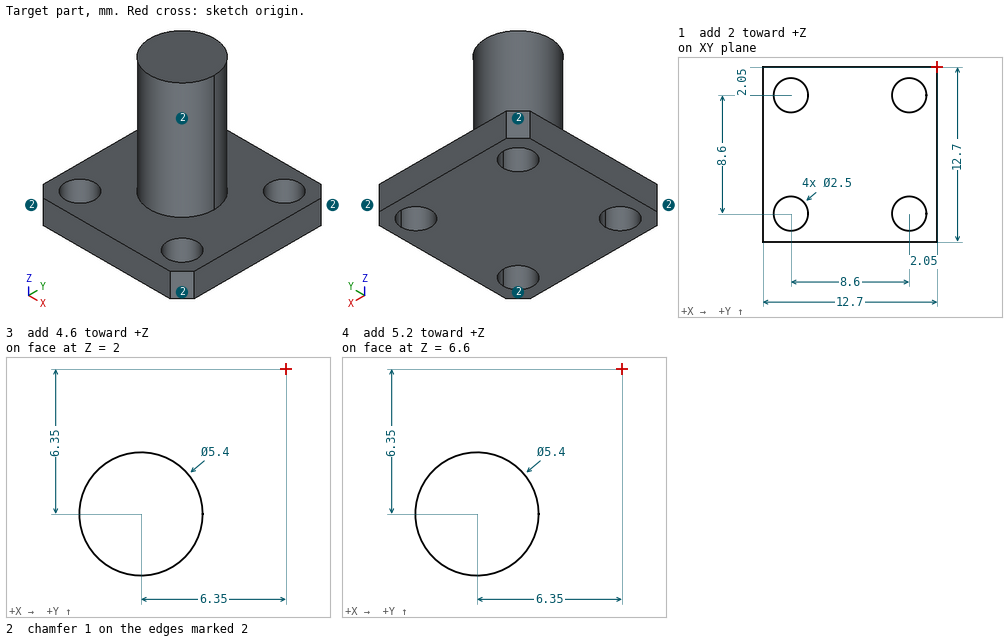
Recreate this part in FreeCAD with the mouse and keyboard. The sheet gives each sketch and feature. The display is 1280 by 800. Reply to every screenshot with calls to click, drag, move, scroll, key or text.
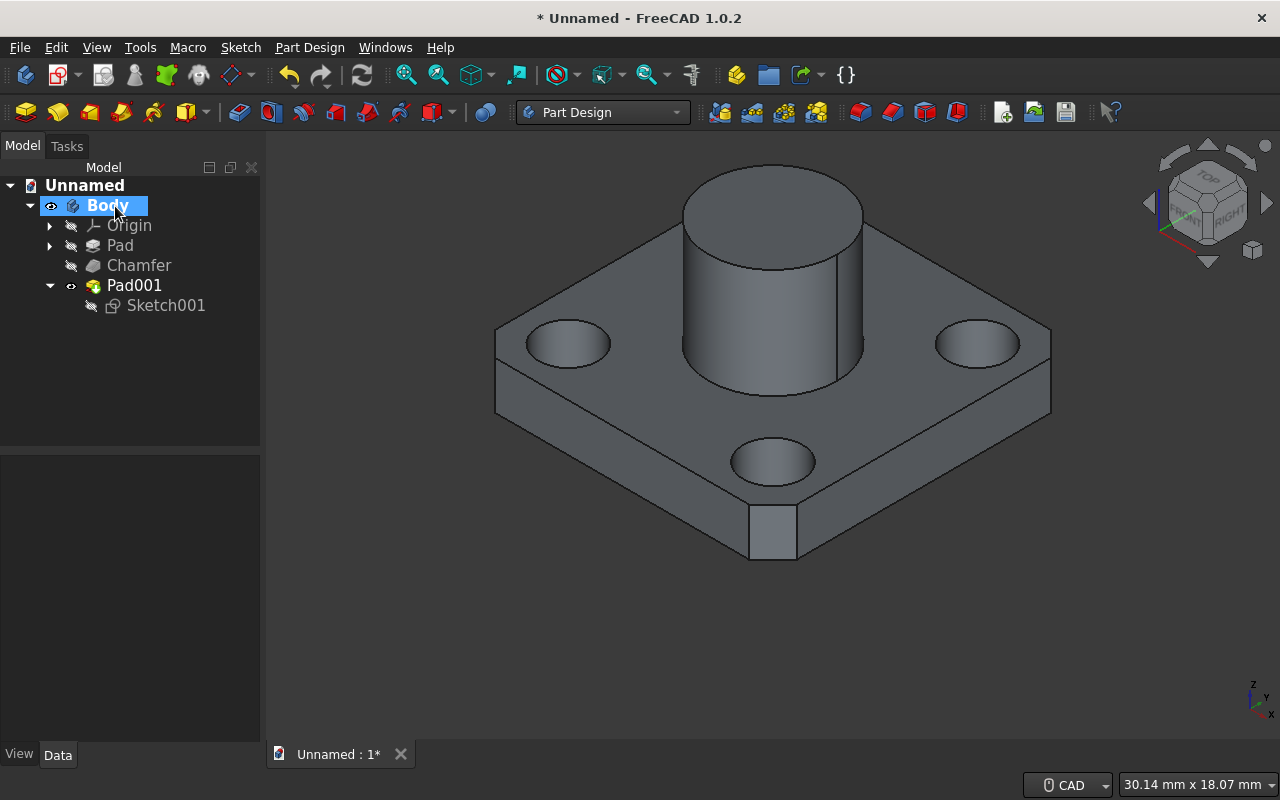
key(v)
key(f)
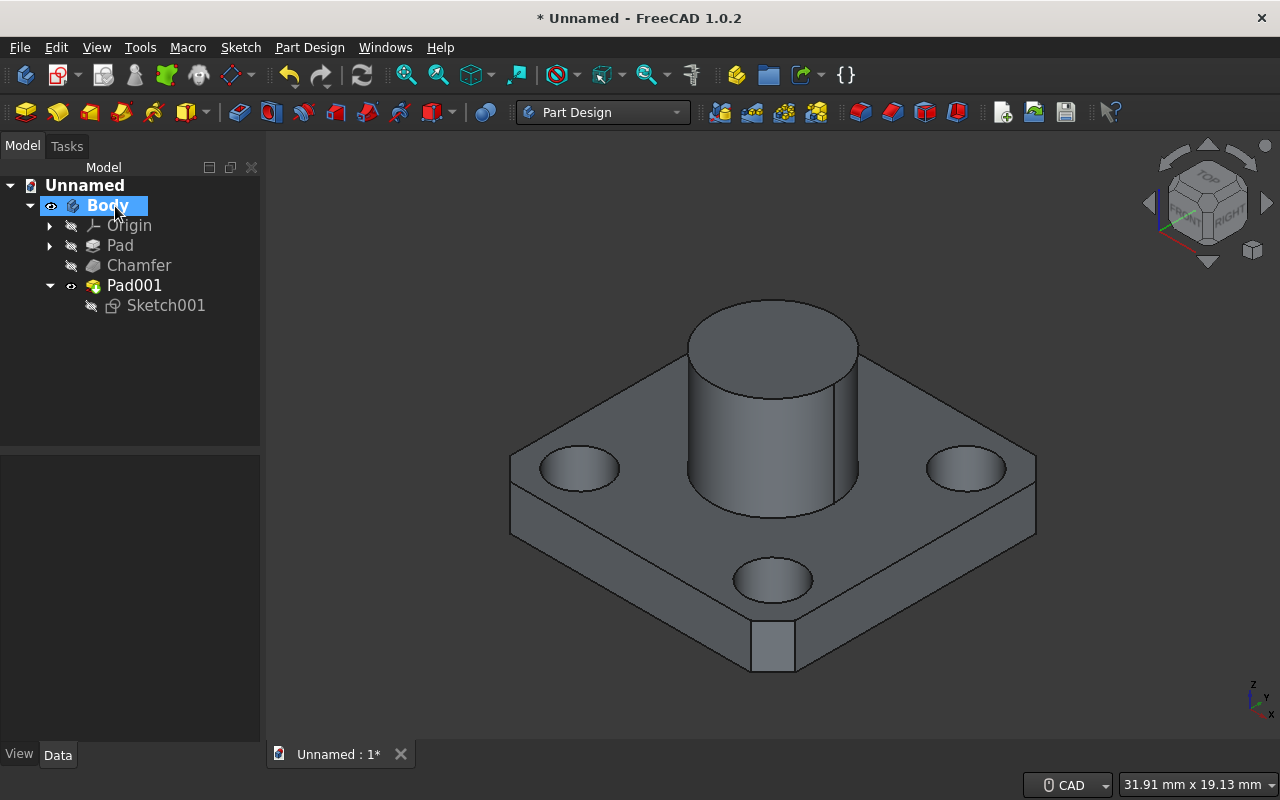
click(773, 348)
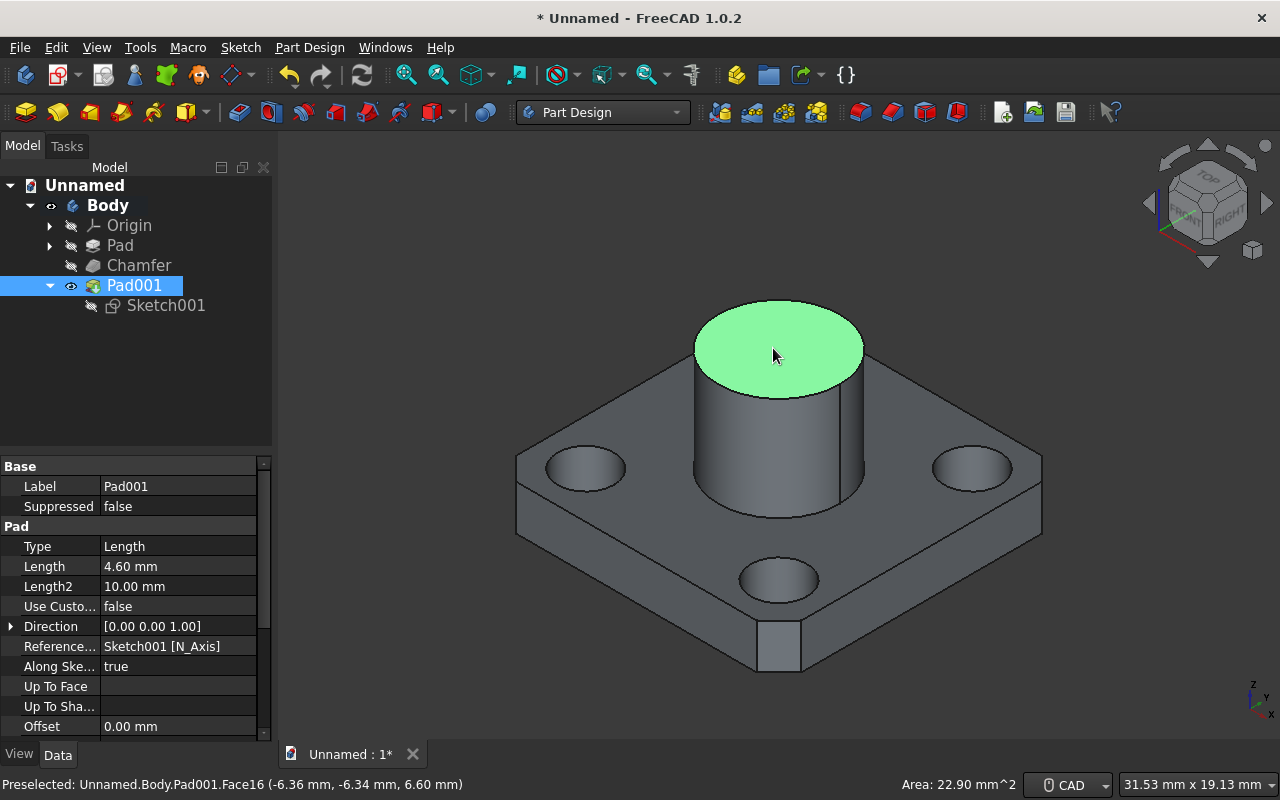
click(58, 76)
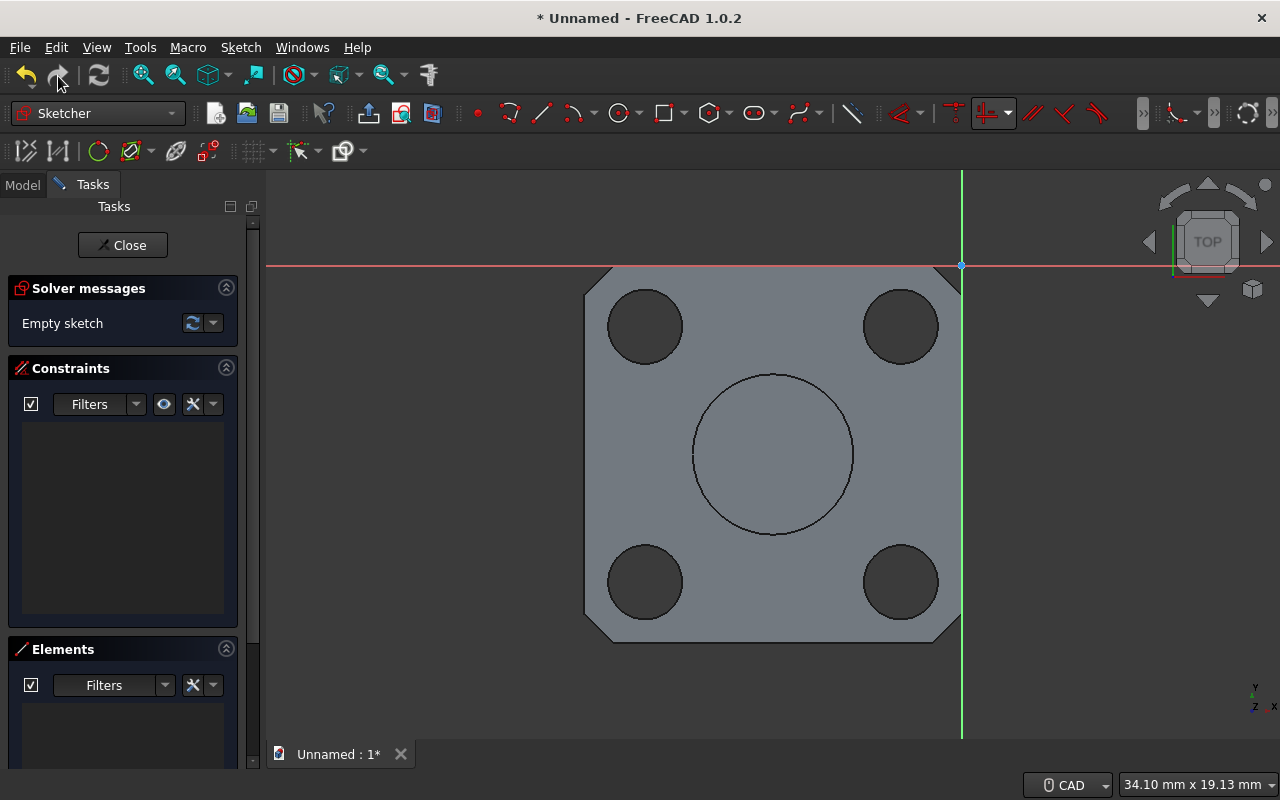
key(g)
key(c)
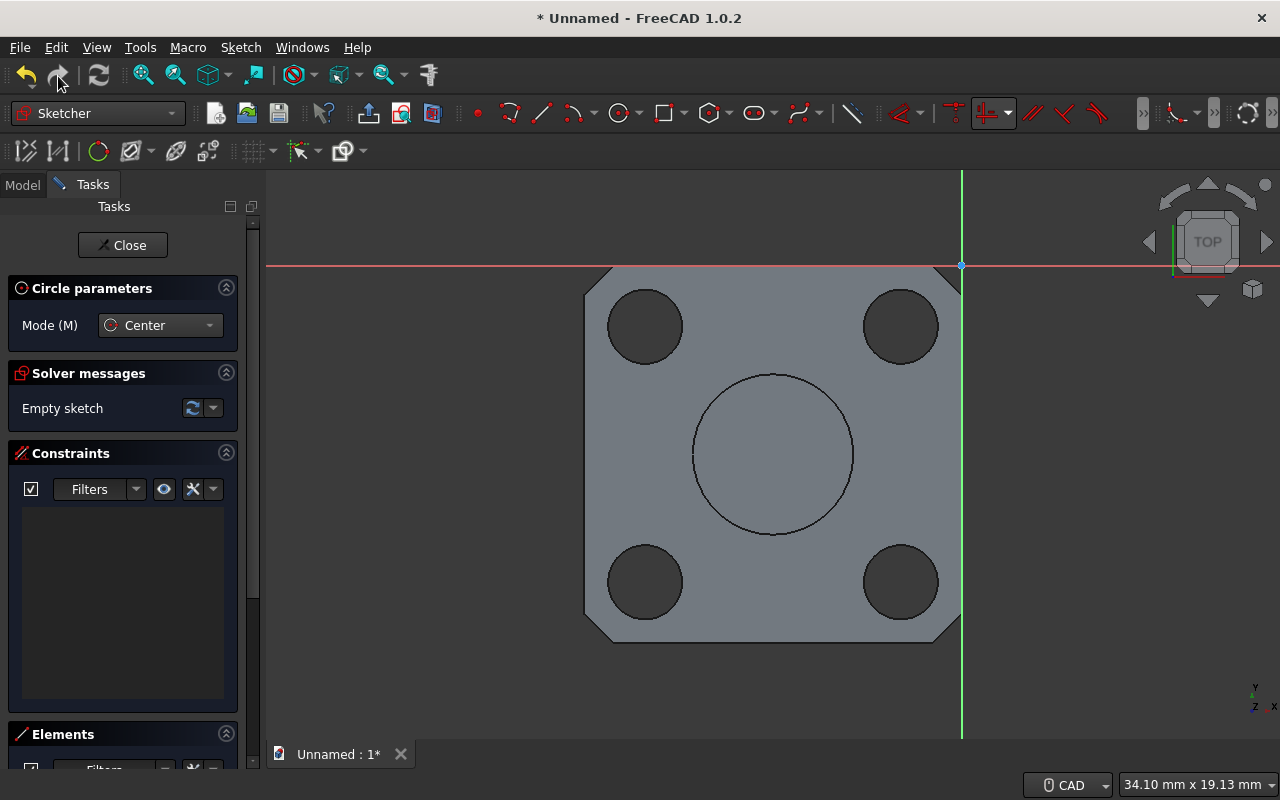
click(773, 455)
move(830, 398)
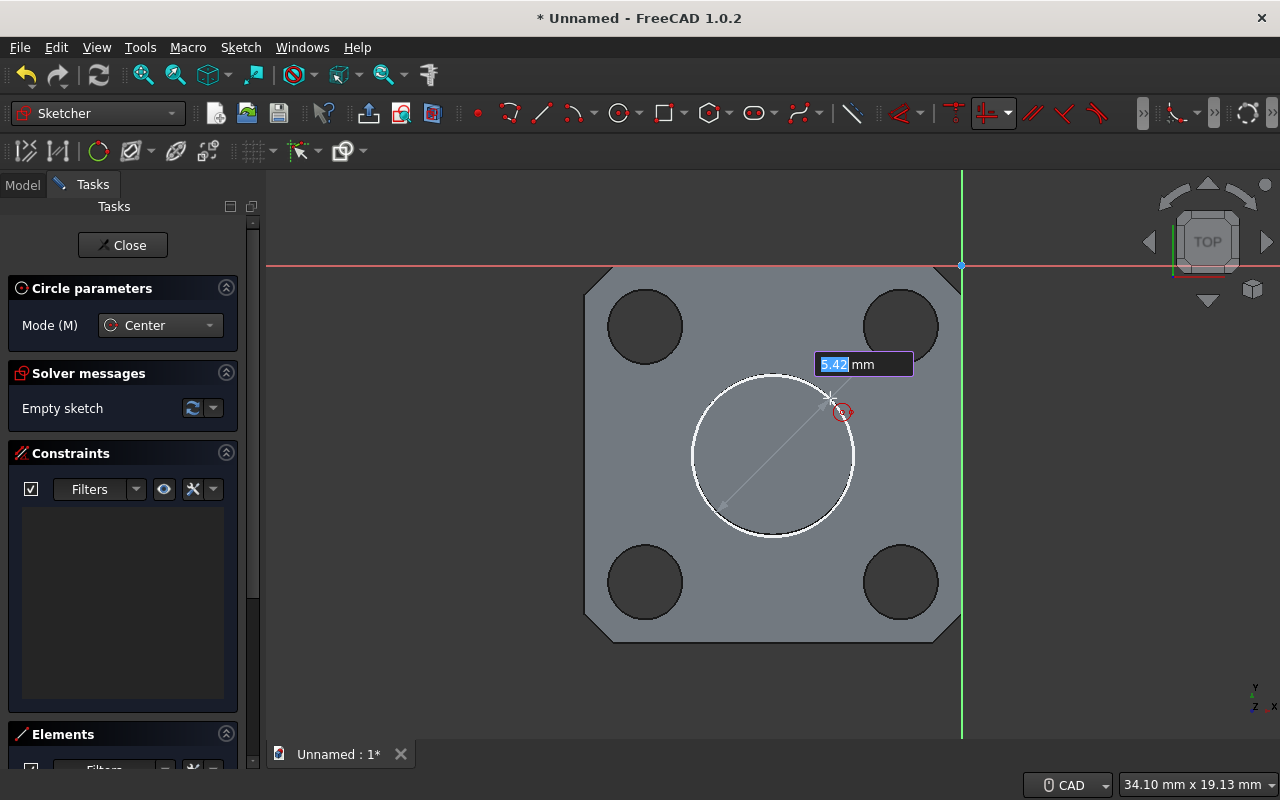
text(5.4)
key(Return)
key(Escape)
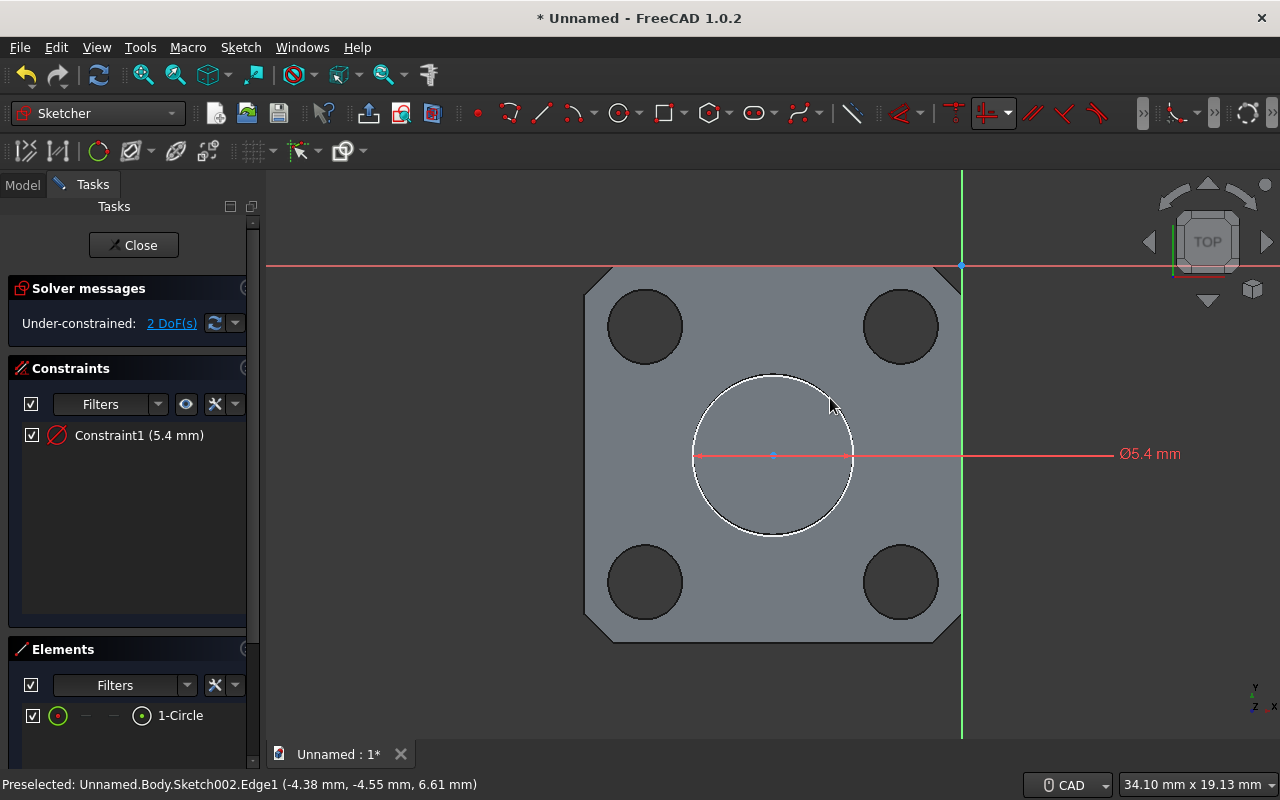
click(900, 114)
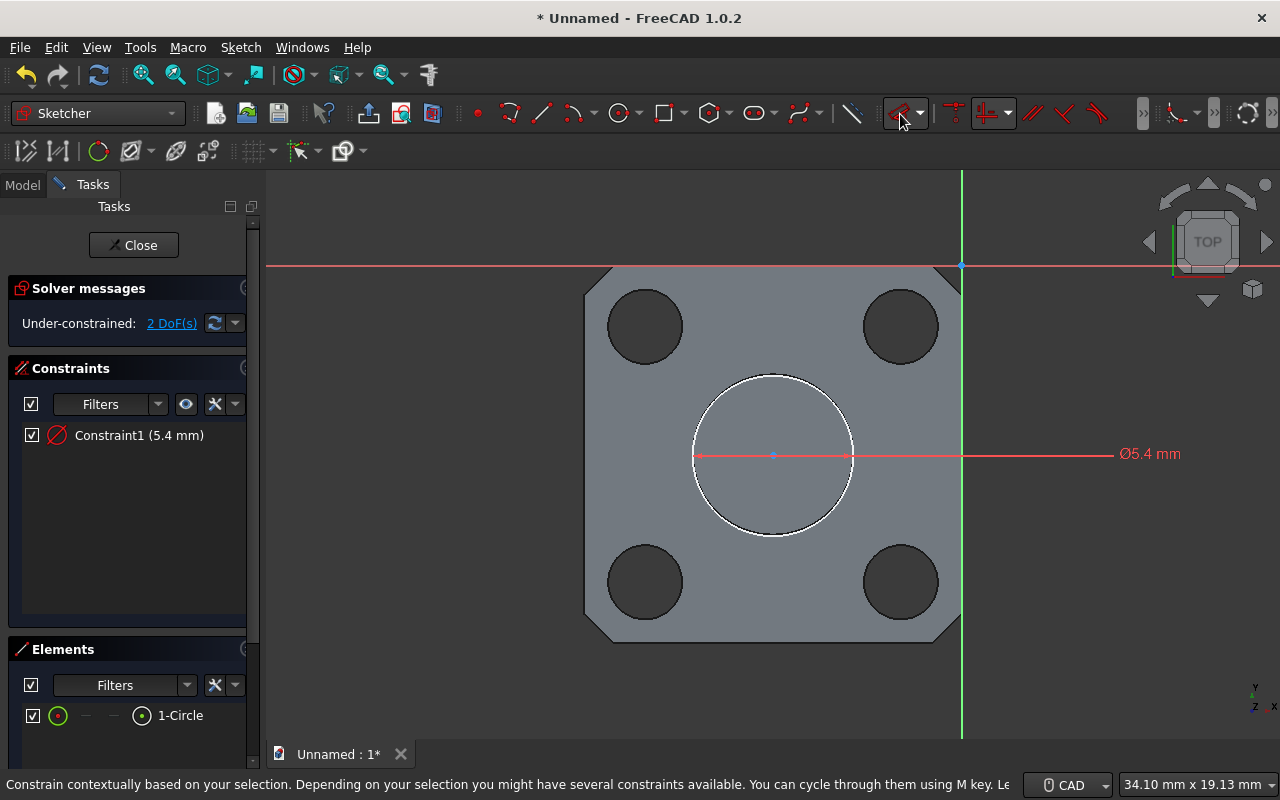
click(773, 456)
click(867, 232)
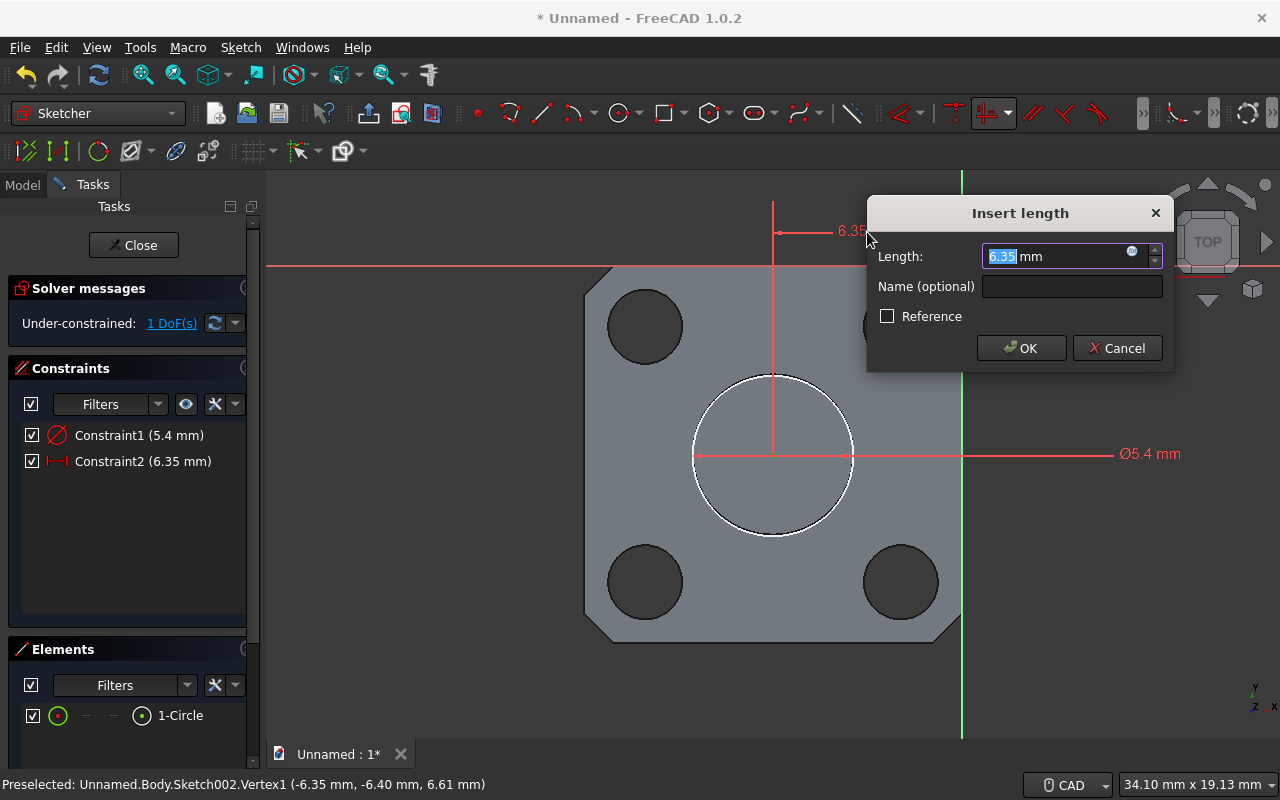
text(6.35)
key(Return)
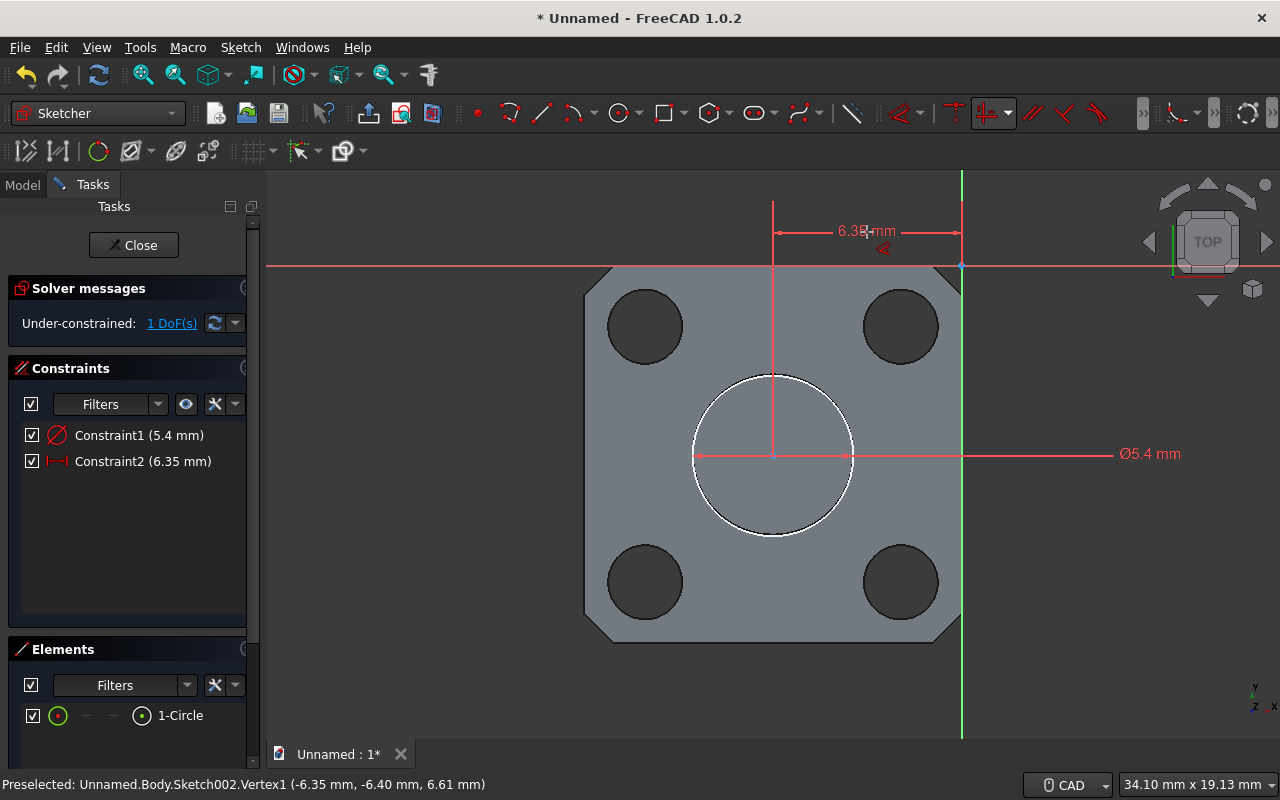
click(773, 456)
click(996, 361)